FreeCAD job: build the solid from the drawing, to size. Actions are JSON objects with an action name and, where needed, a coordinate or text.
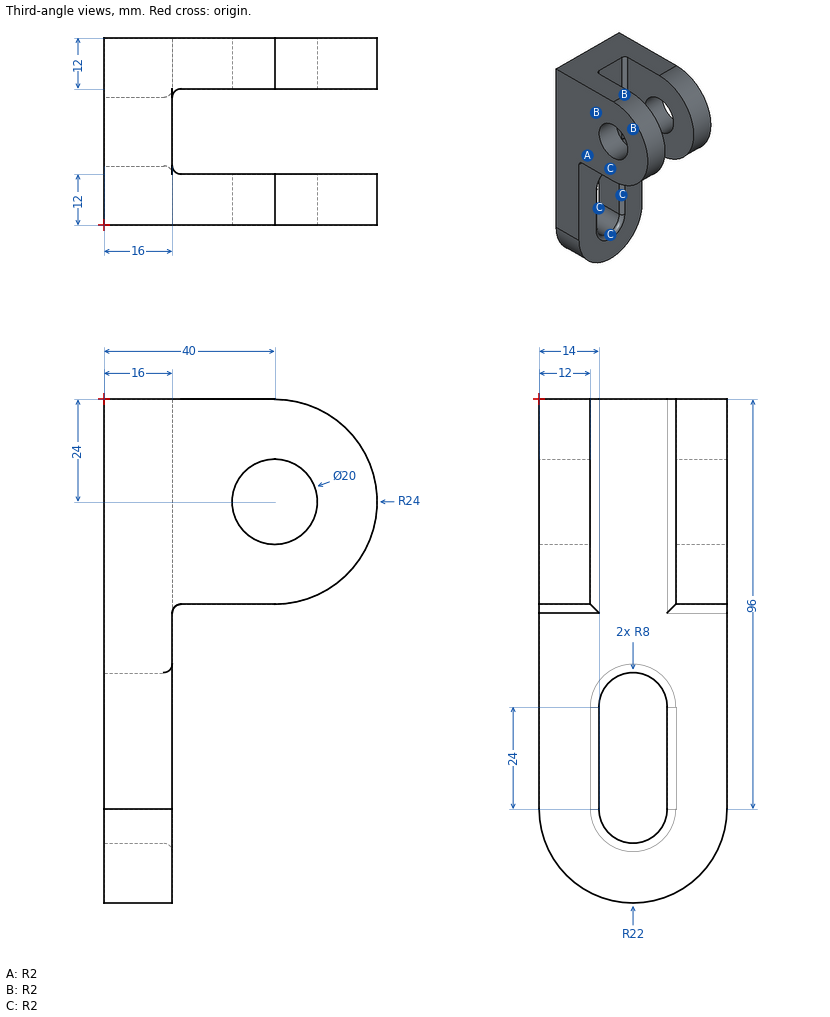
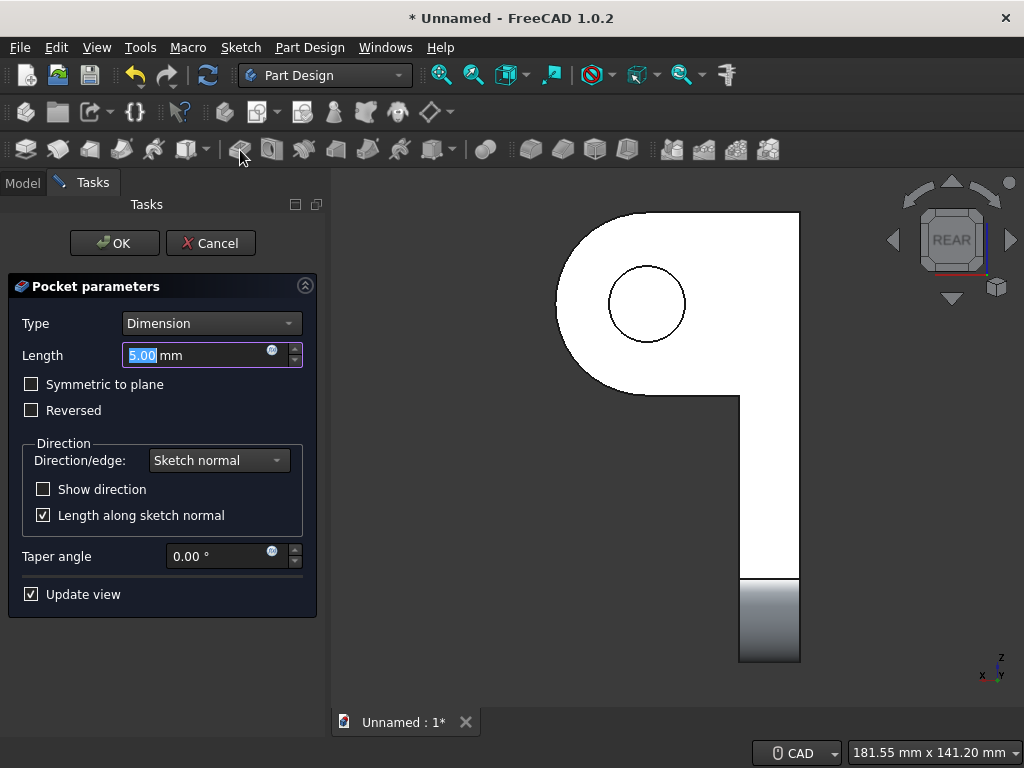
{"action": "type", "text": "12"}
{"action": "key", "text": "Tab"}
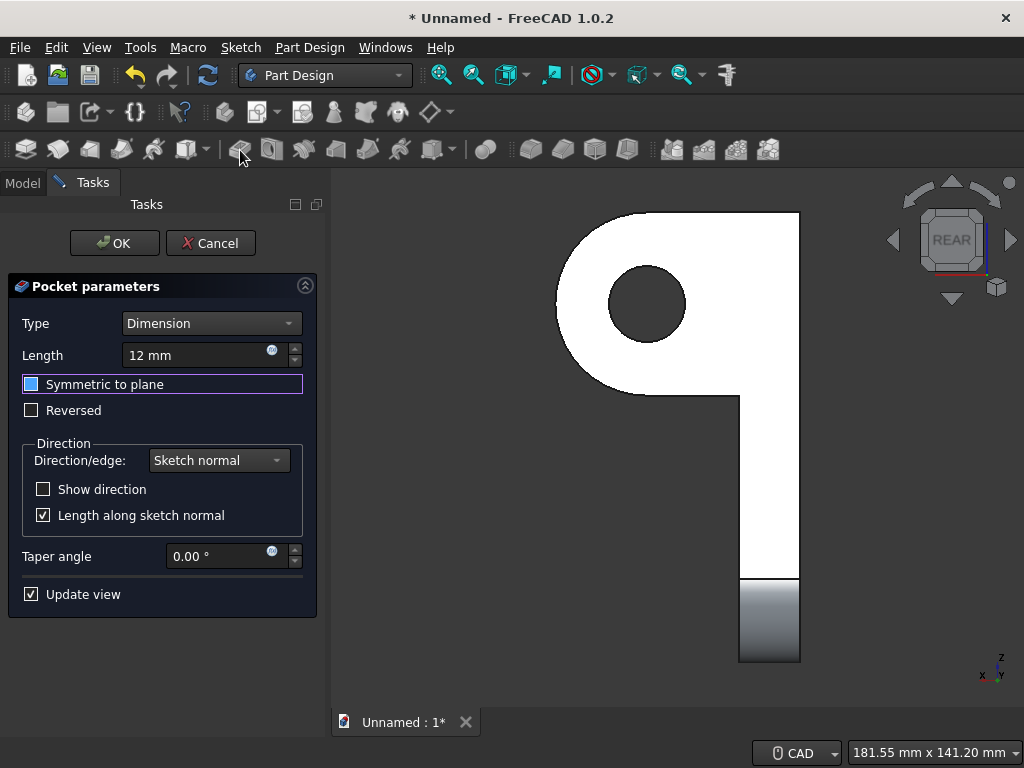
{"action": "left_click", "coordinate": [115, 243]}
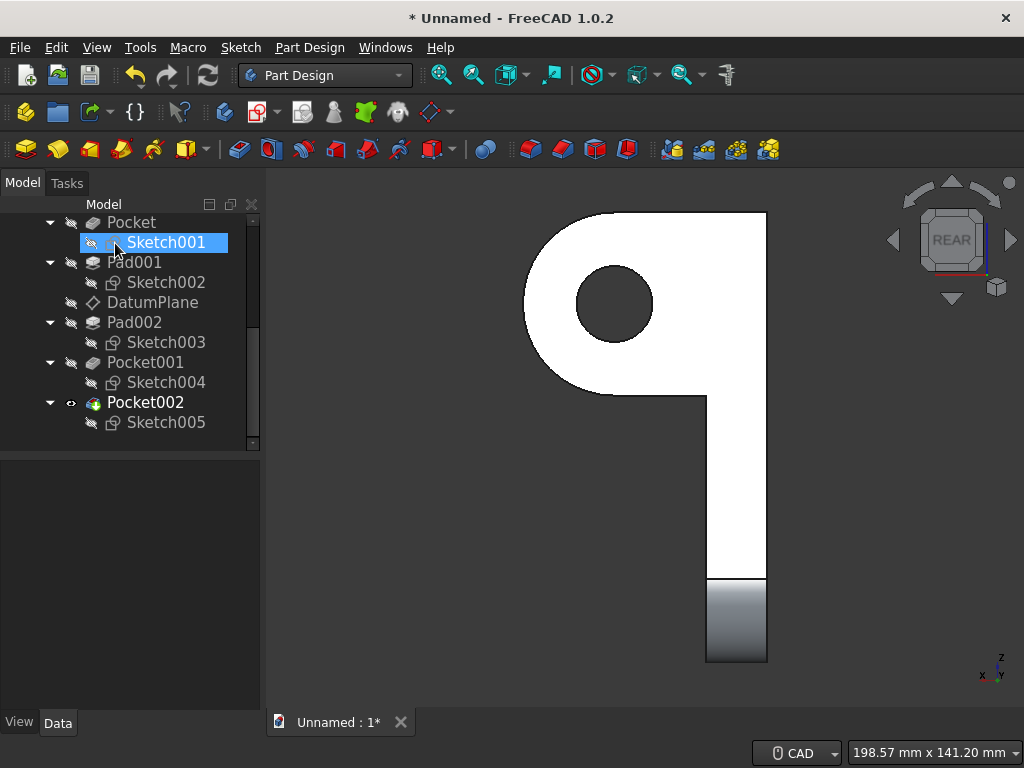
{"action": "key", "text": "0"}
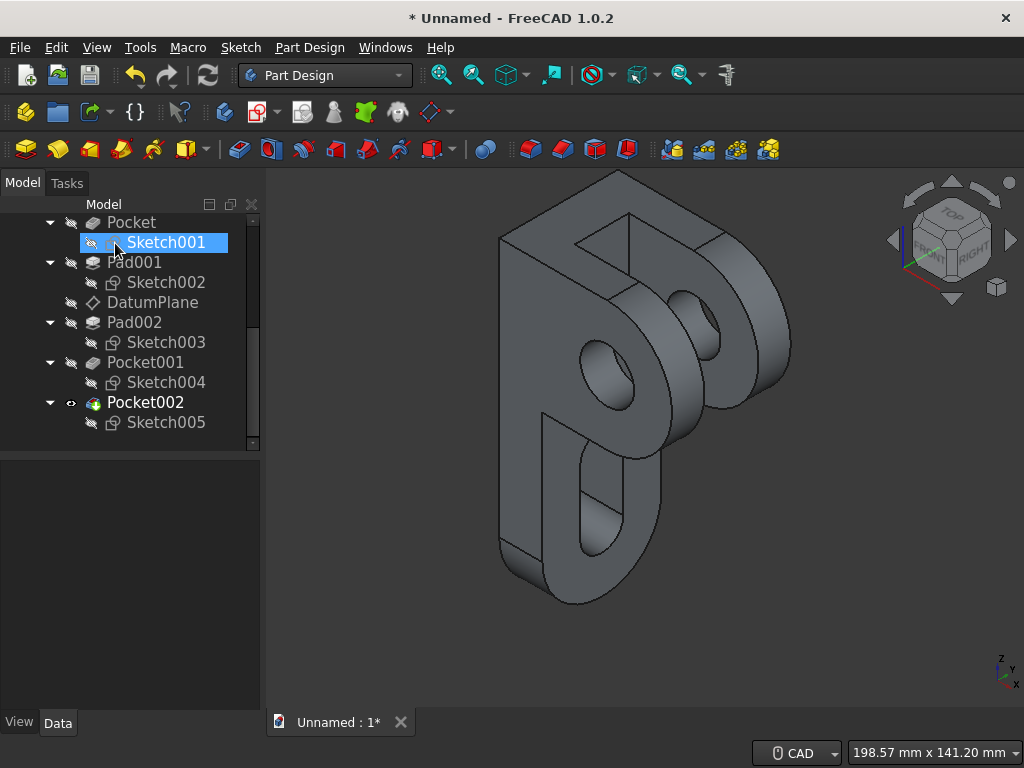
{"action": "key", "text": "2"}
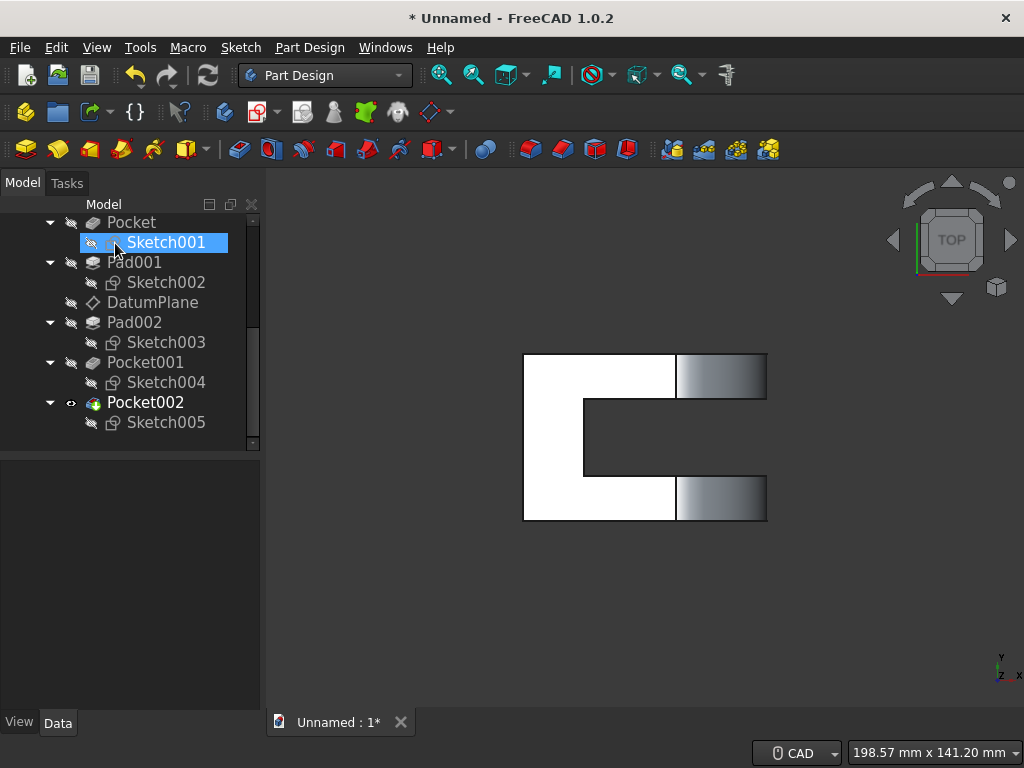
{"action": "left_click", "coordinate": [442, 76]}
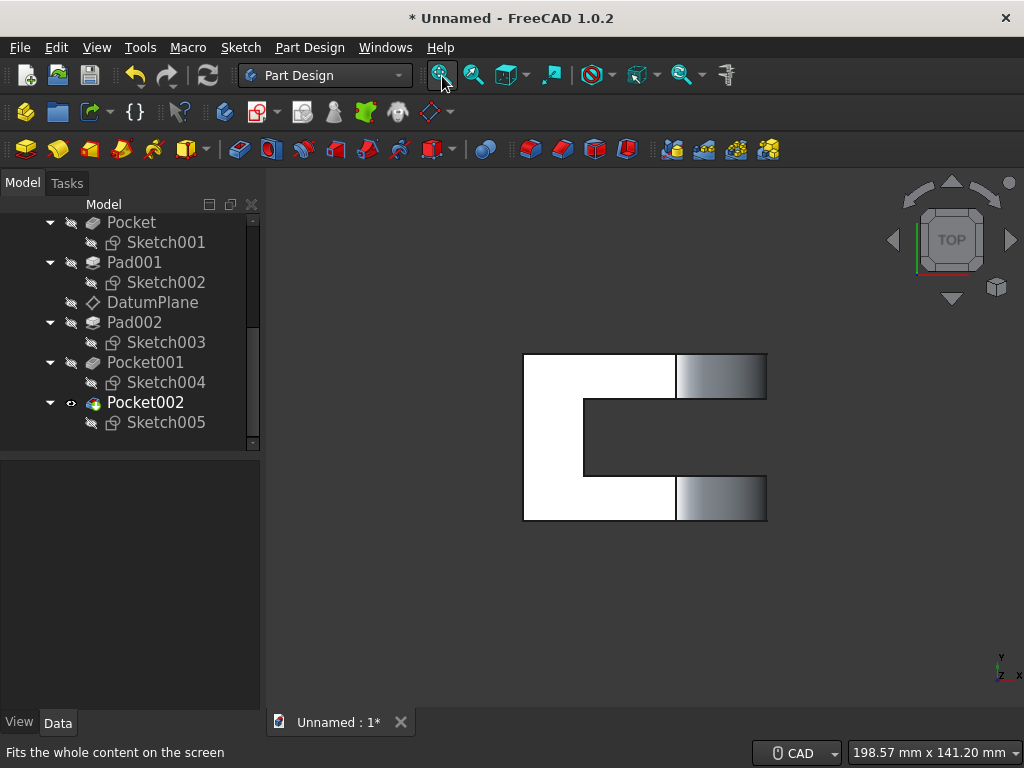
{"action": "key", "text": "1"}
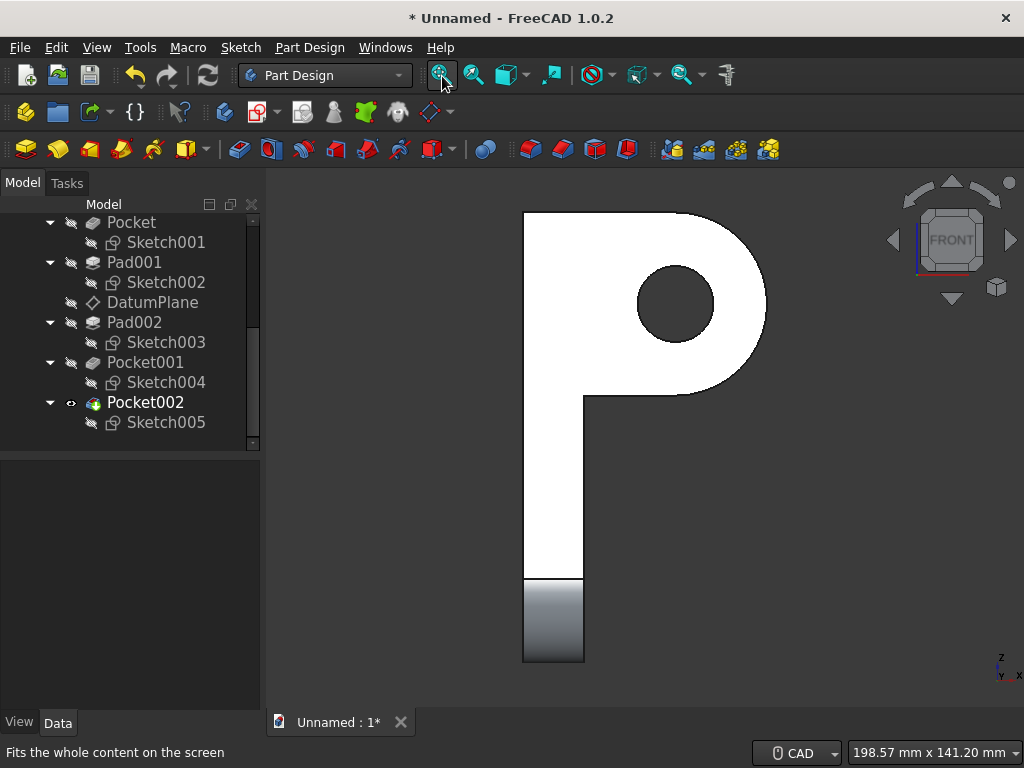
{"action": "key", "text": "3"}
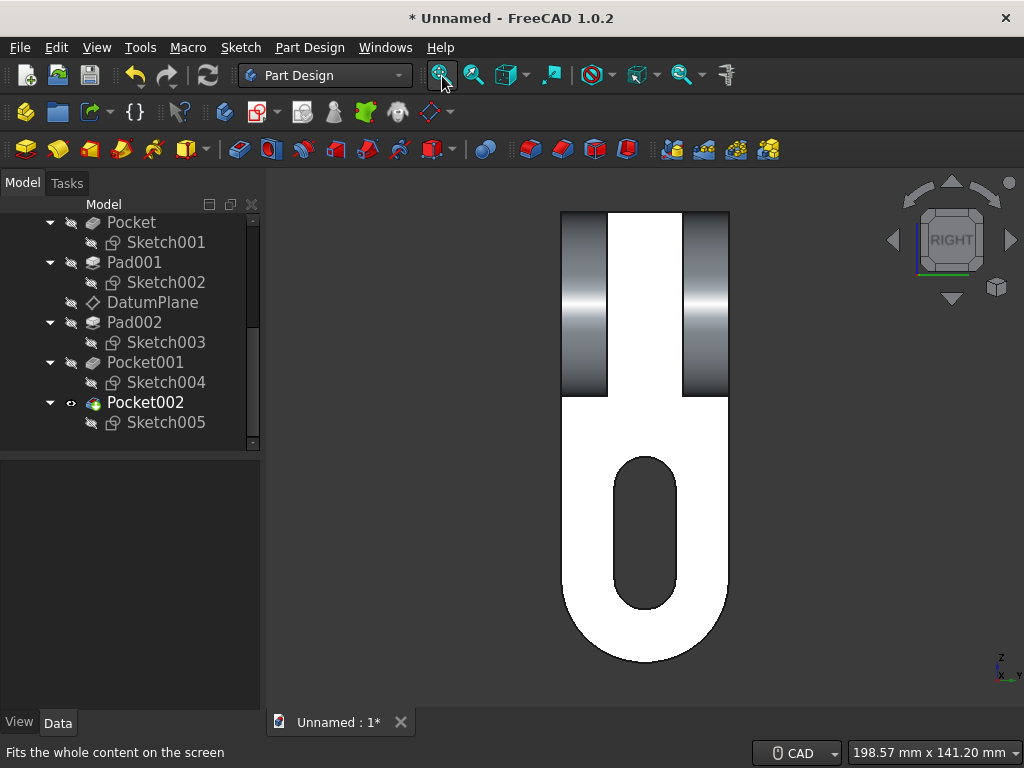
{"action": "key", "text": "5"}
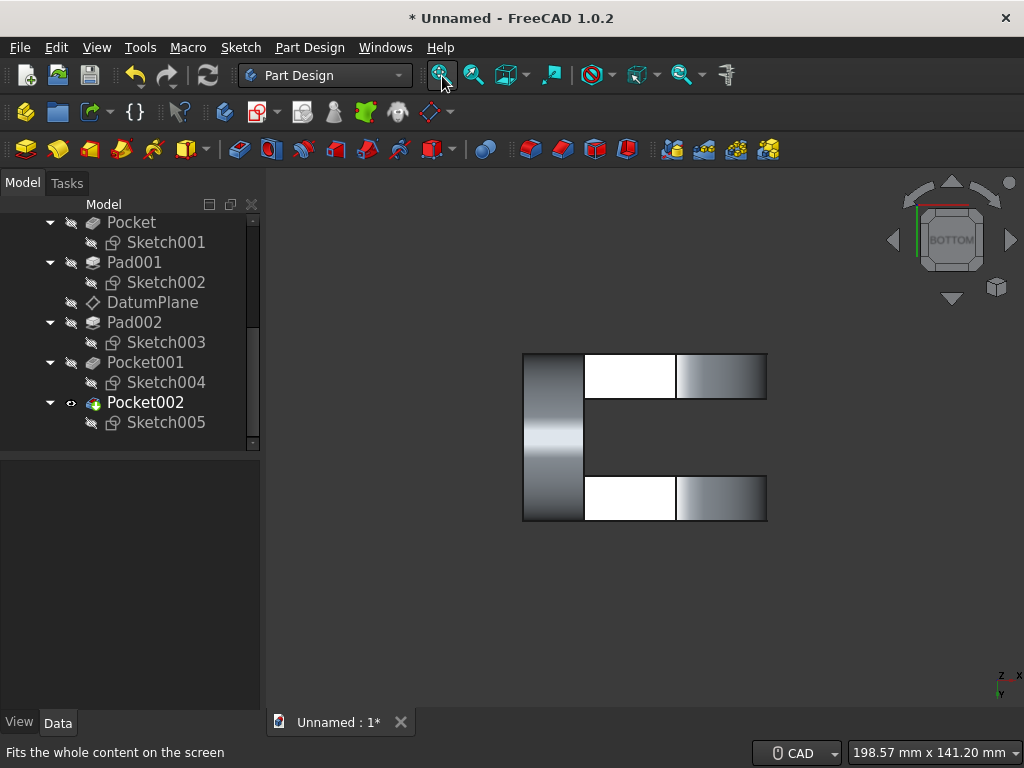
{"action": "left_click", "coordinate": [442, 76]}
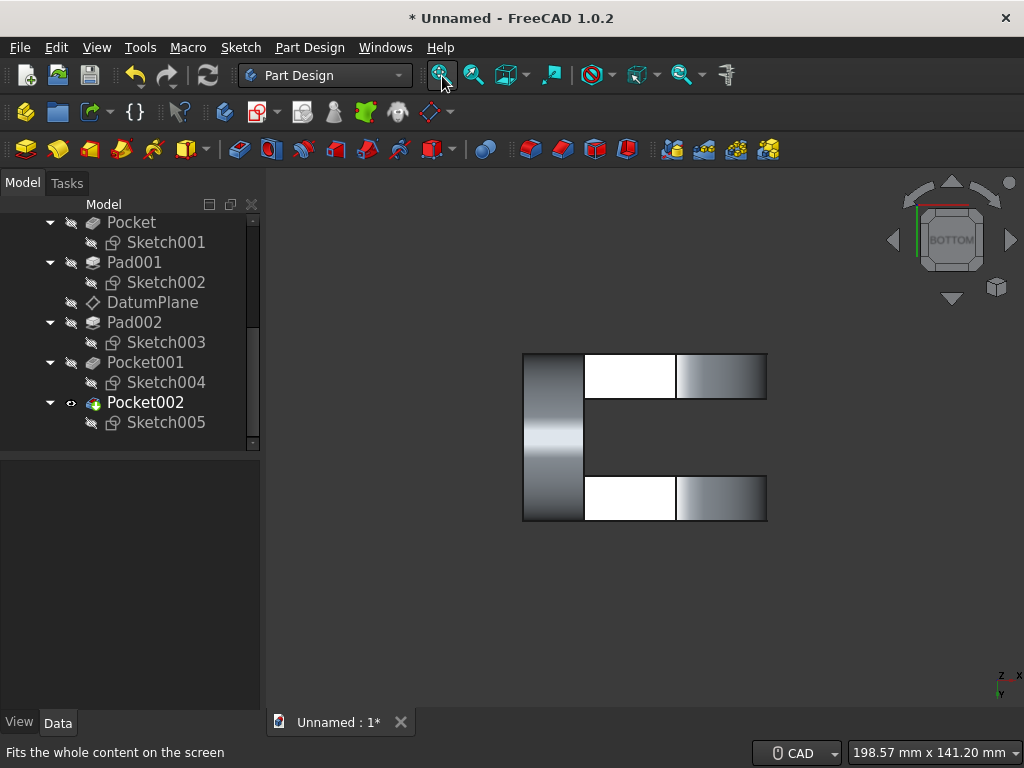
{"action": "key", "text": "4"}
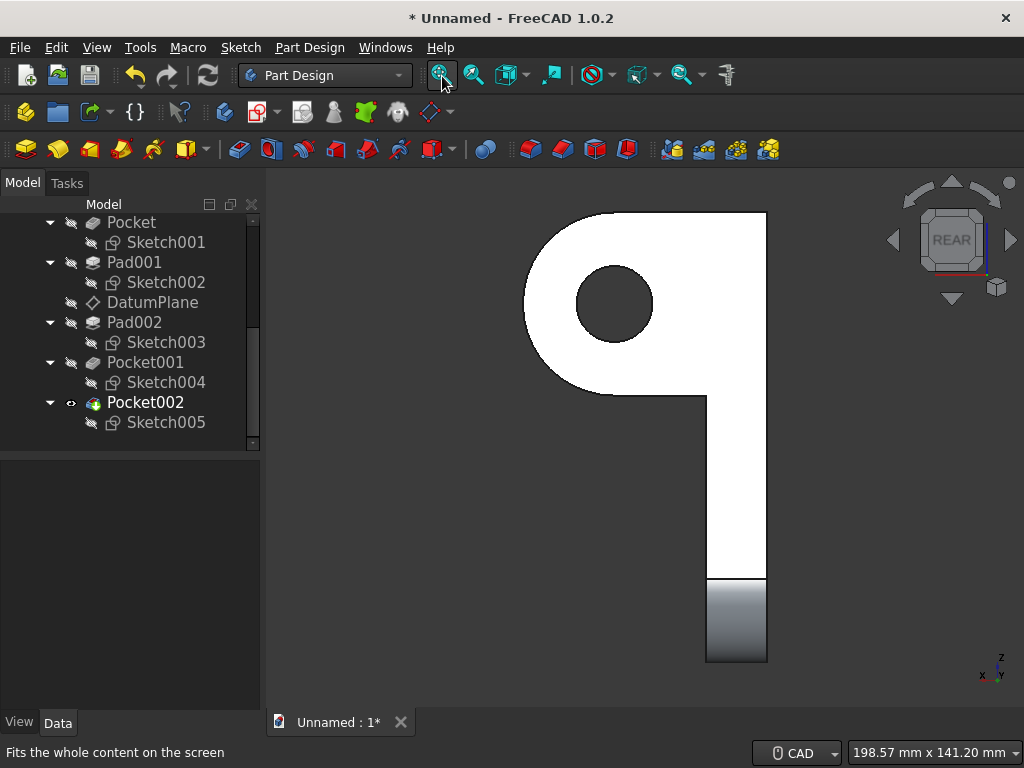
{"action": "key", "text": "6"}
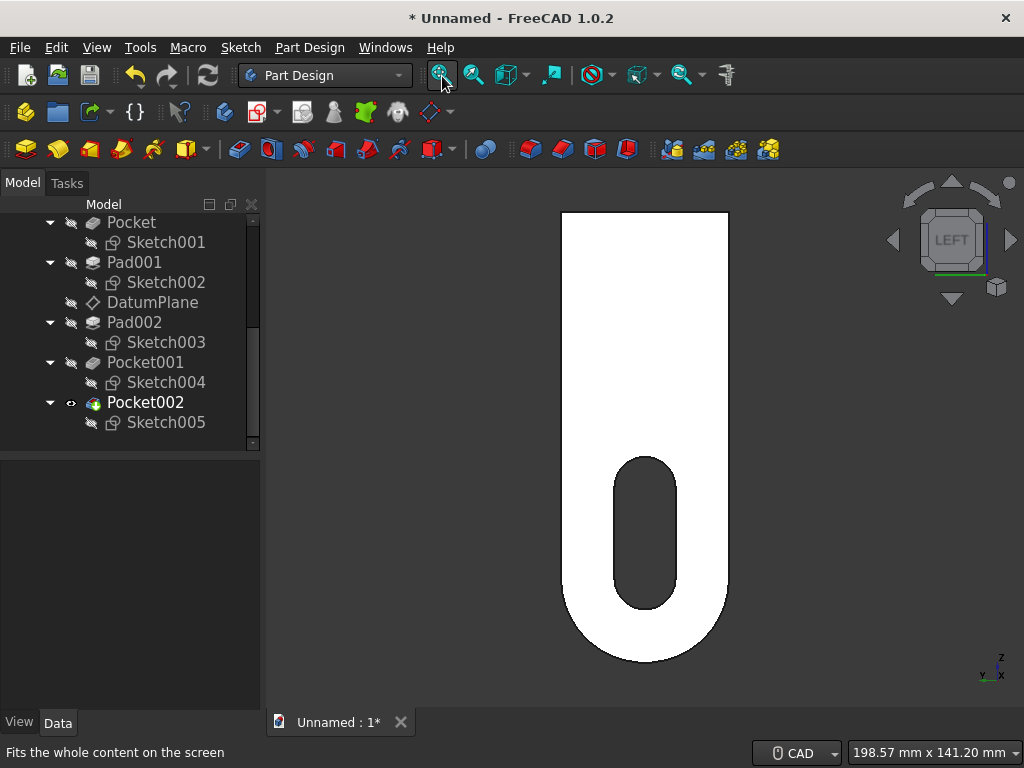
{"action": "key", "text": "v 3"}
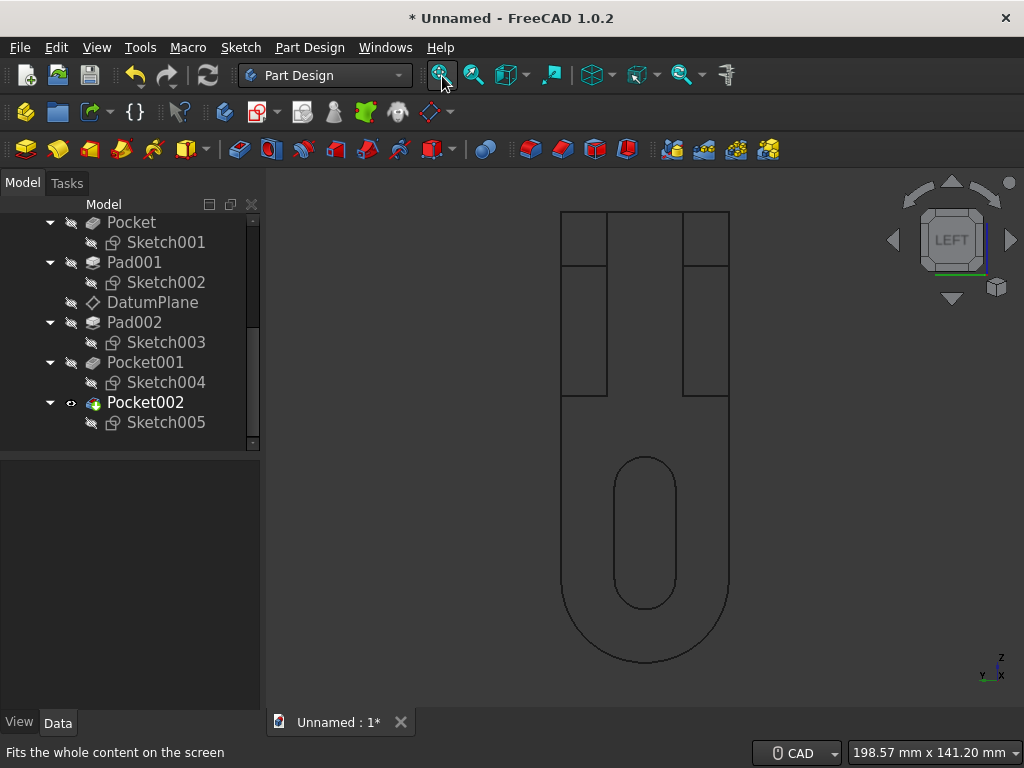
{"action": "key", "text": "0"}